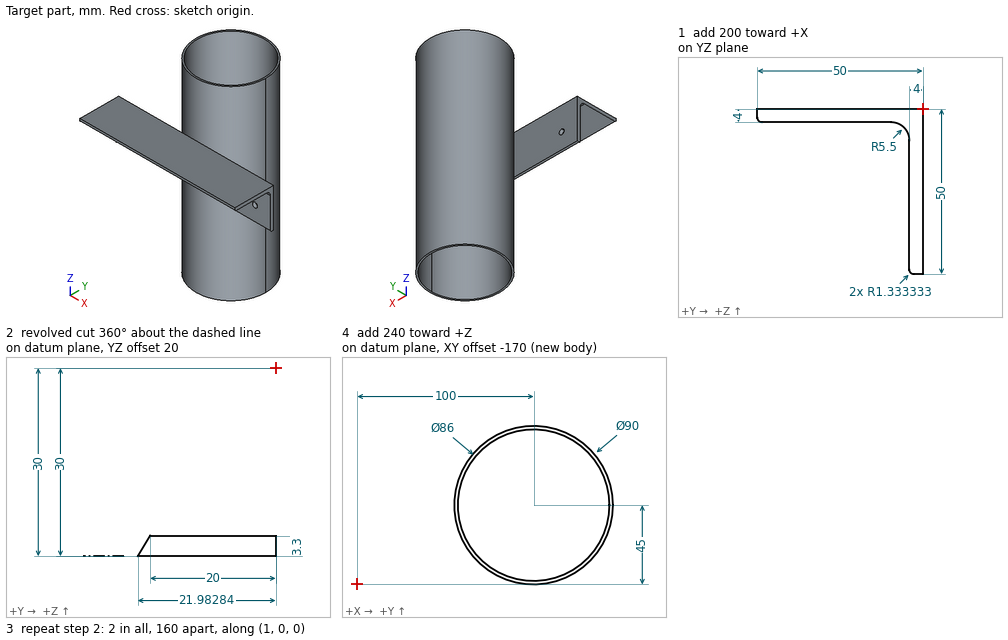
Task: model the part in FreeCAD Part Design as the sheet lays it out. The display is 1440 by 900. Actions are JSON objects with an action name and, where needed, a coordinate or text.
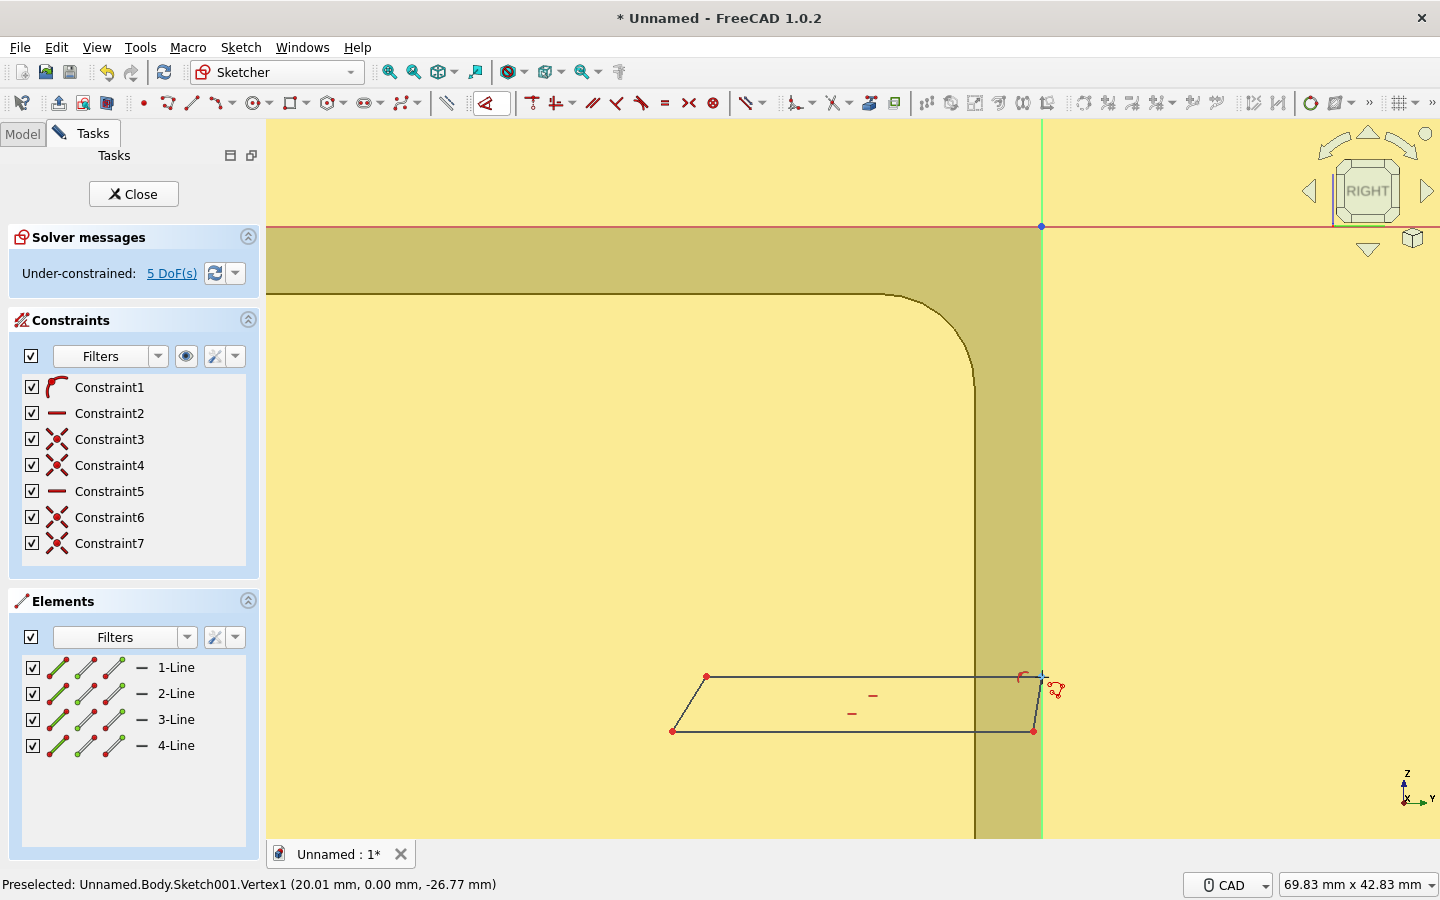
{"action": "left_click", "coordinate": [192, 104]}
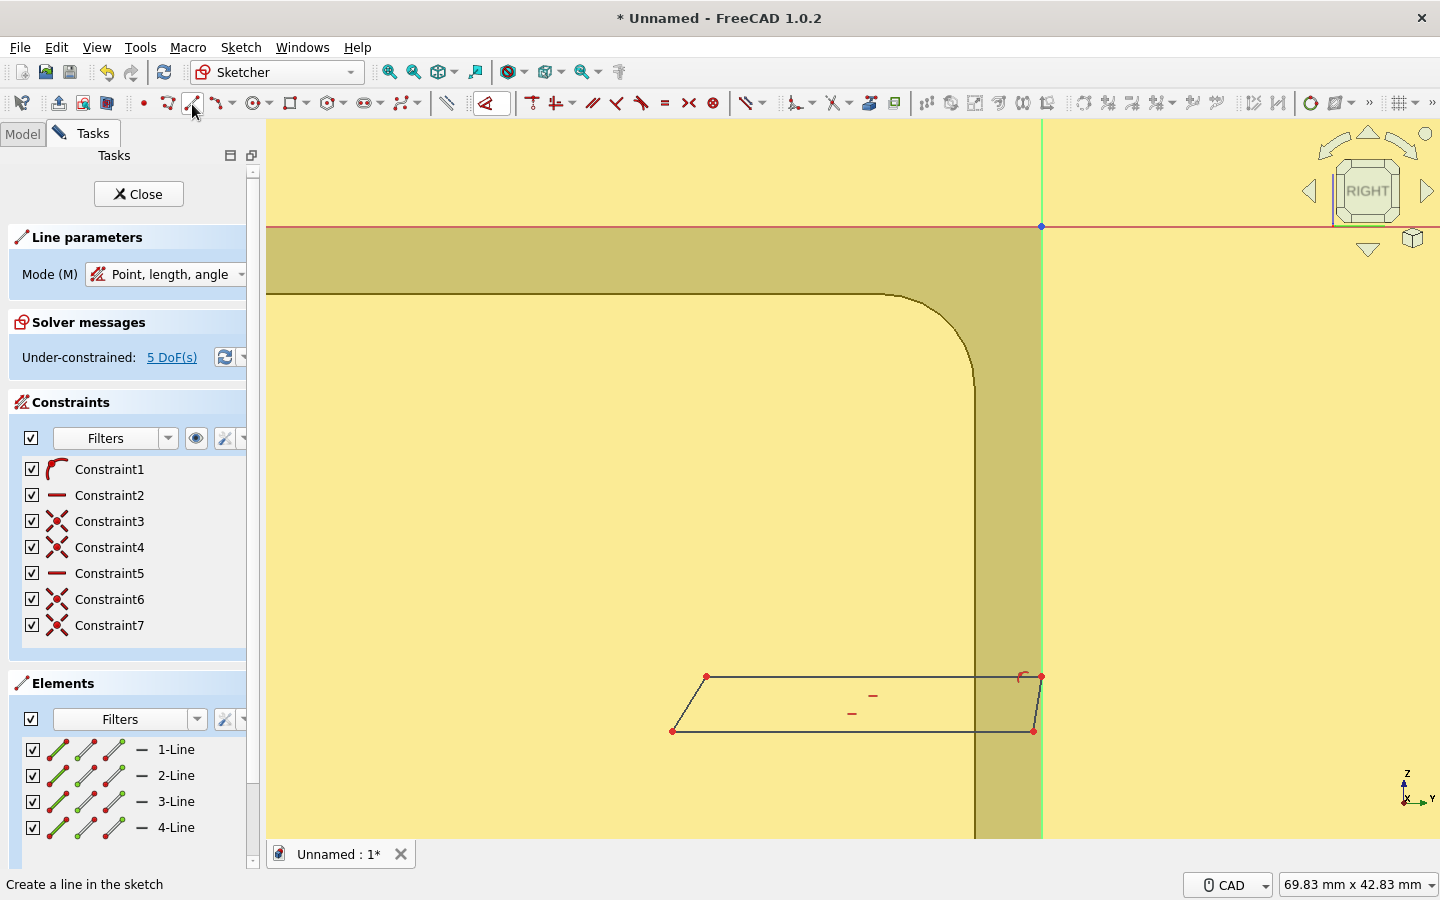
{"action": "left_click", "coordinate": [635, 731]}
{"action": "left_click", "coordinate": [524, 731]}
{"action": "key", "text": "Escape"}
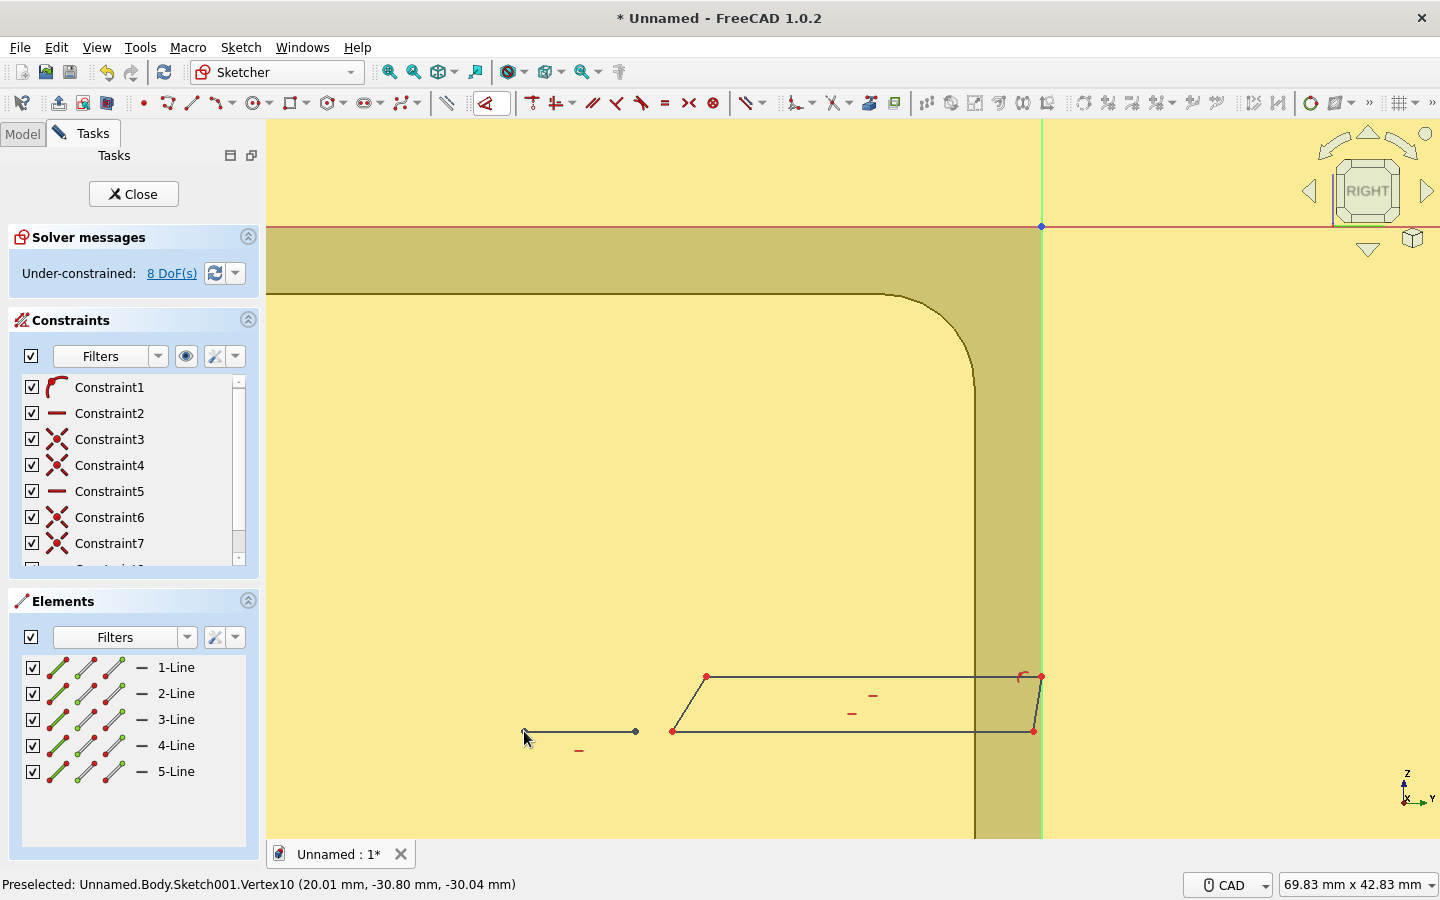
{"action": "left_click", "coordinate": [602, 732]}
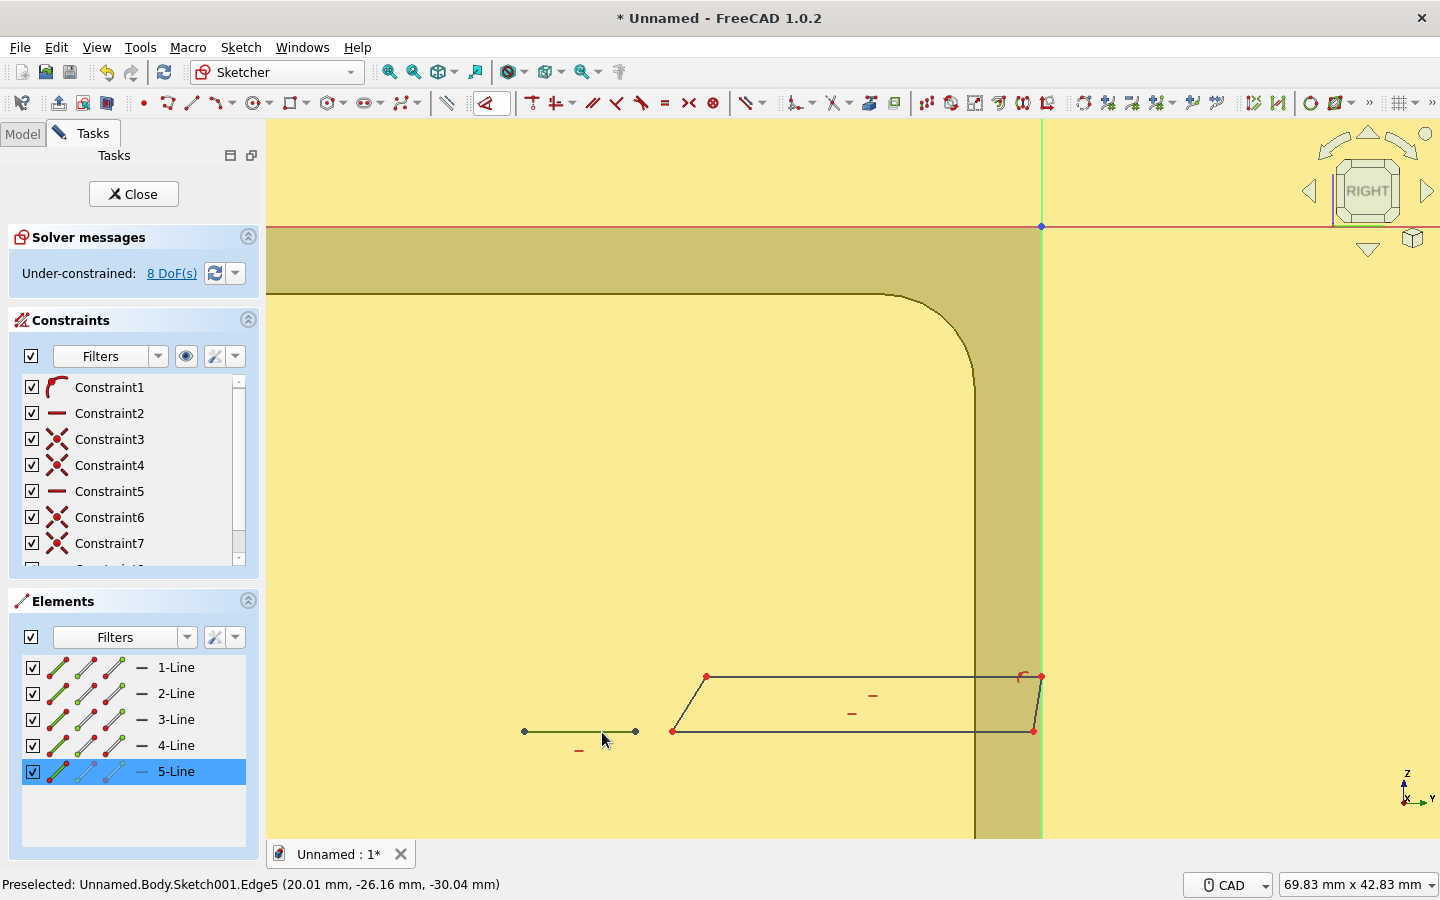
{"action": "left_click", "coordinate": [448, 104]}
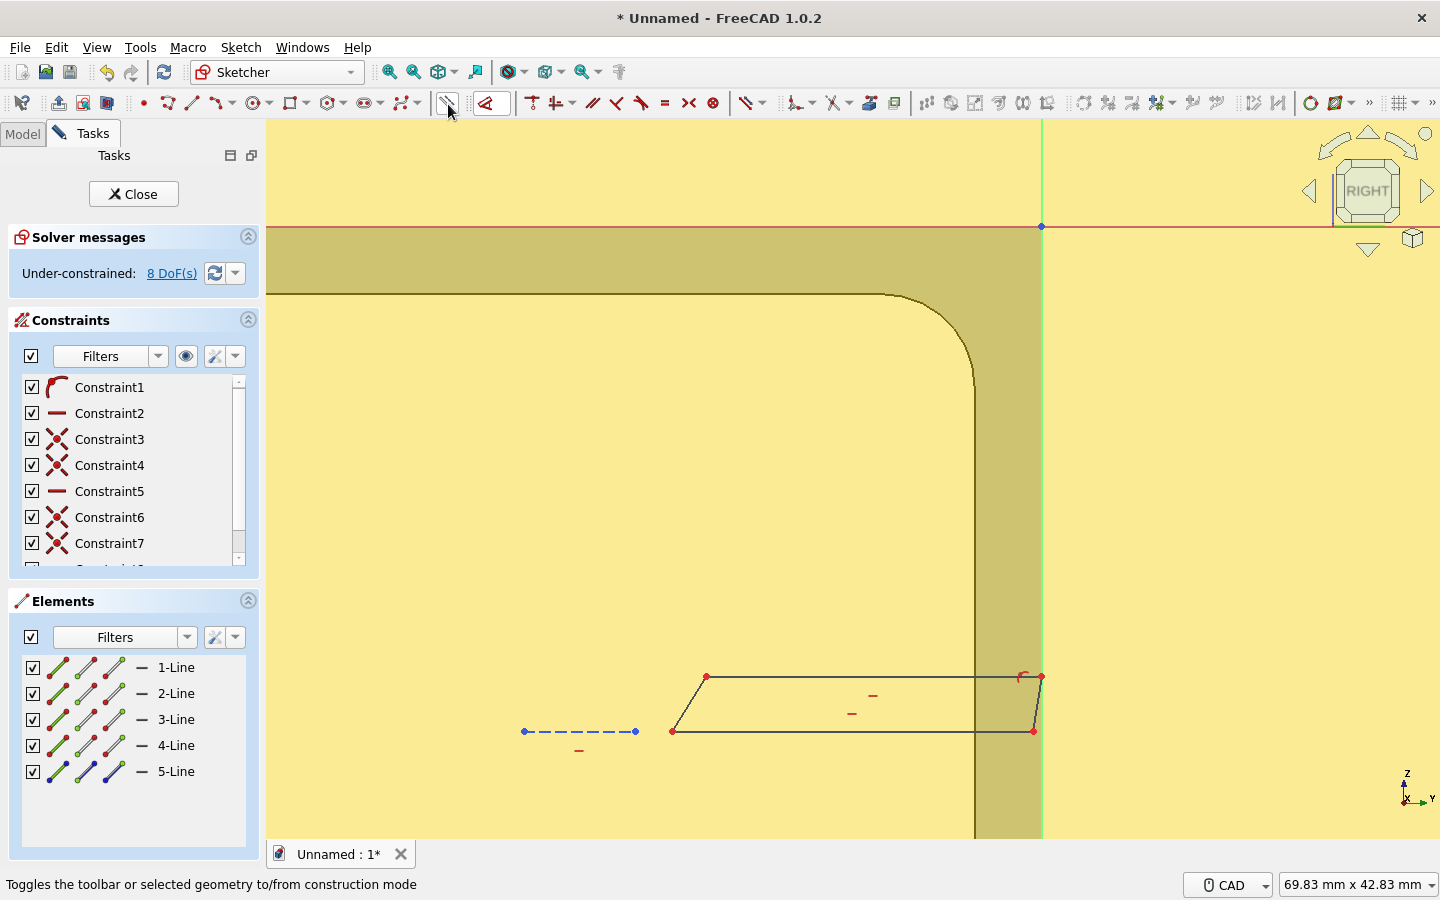
{"action": "left_click", "coordinate": [1039, 694]}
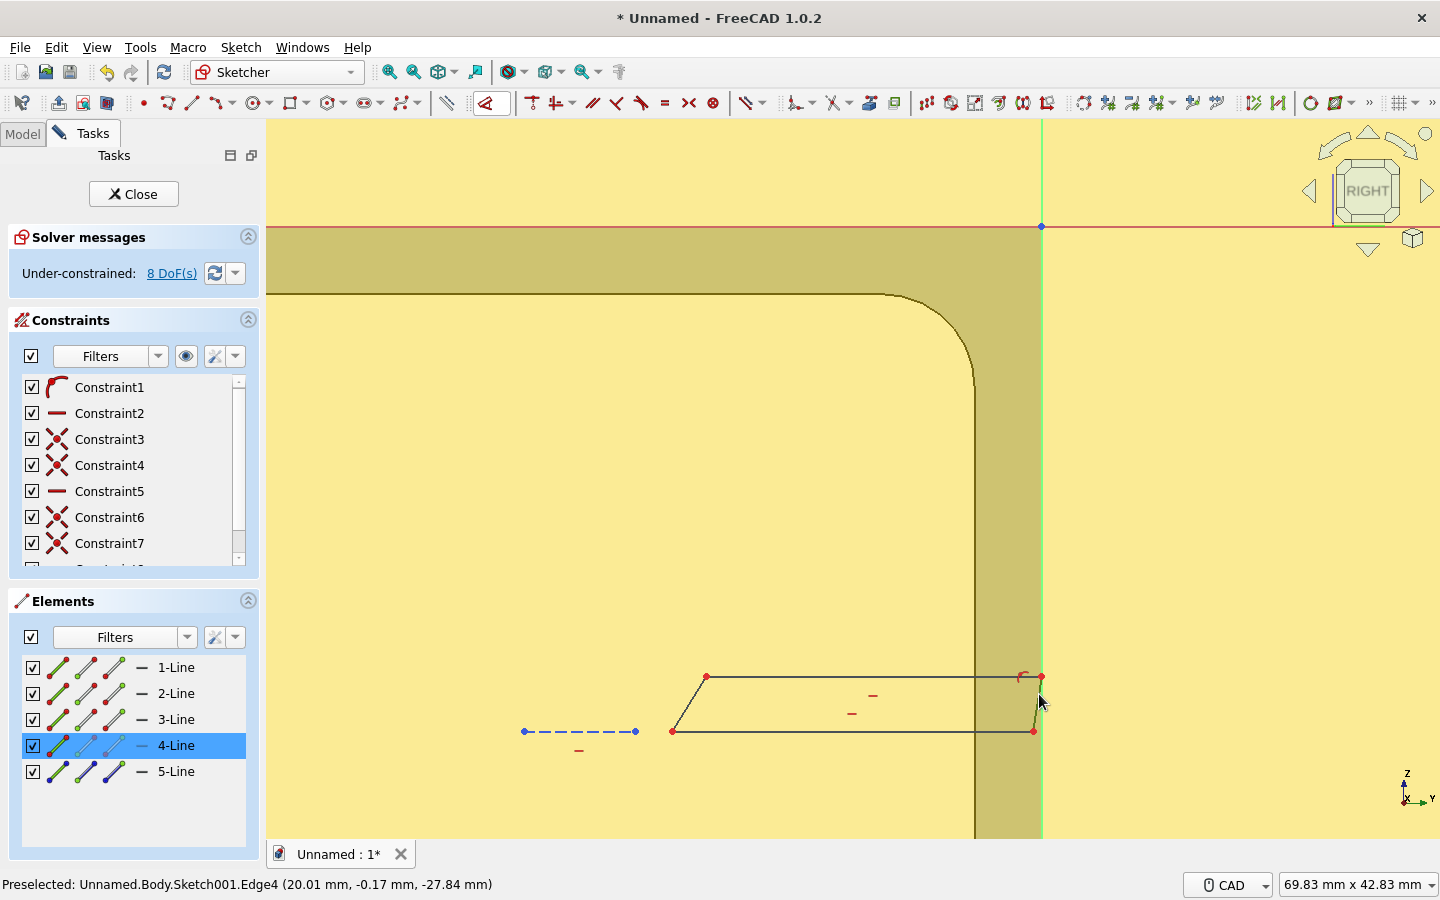
{"action": "left_click", "coordinate": [574, 104]}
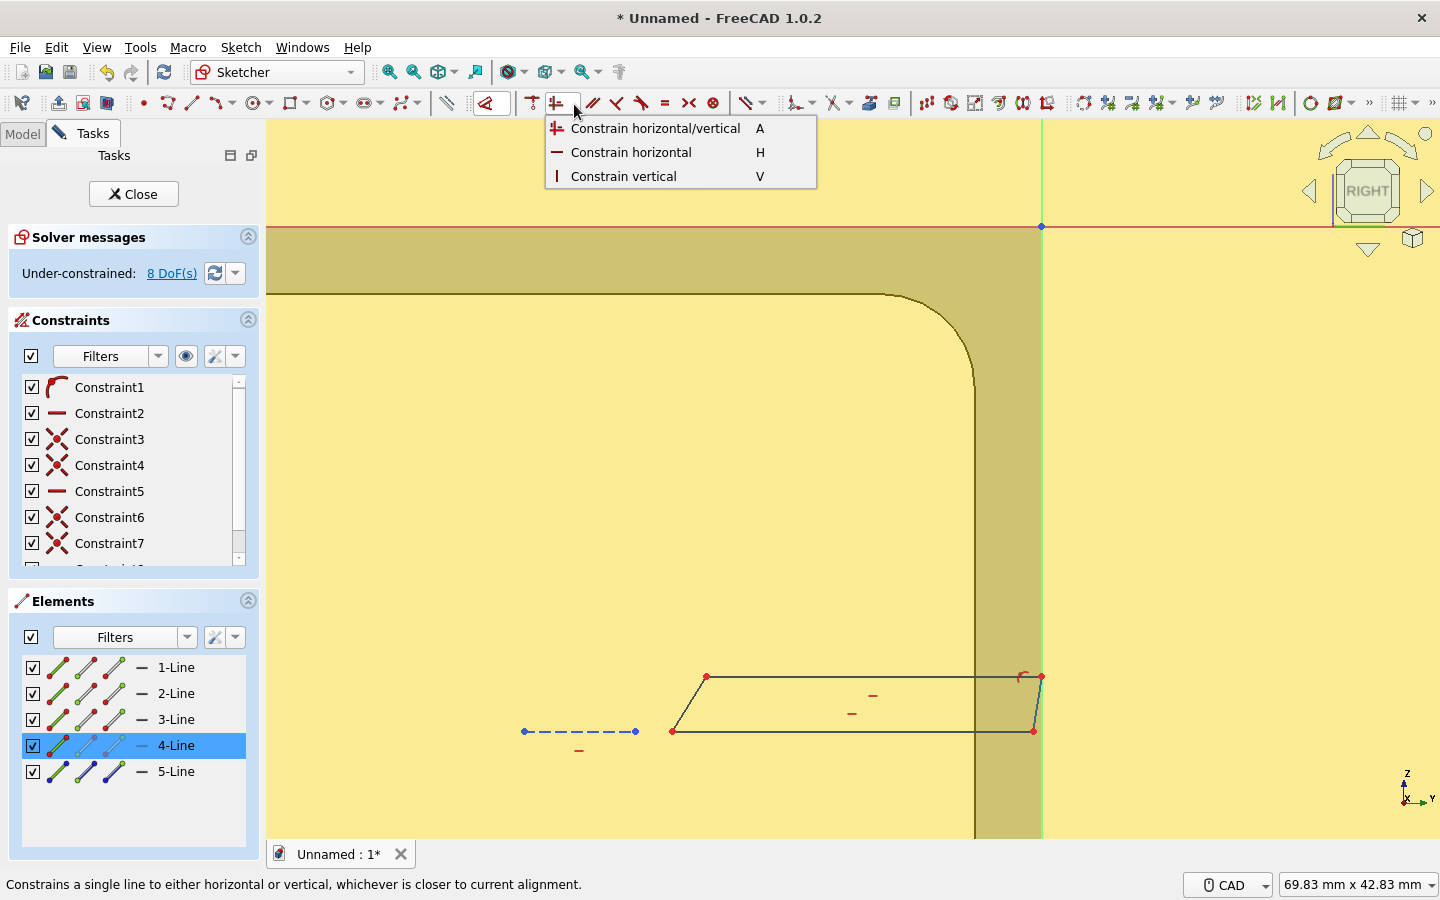
{"action": "left_click", "coordinate": [681, 176]}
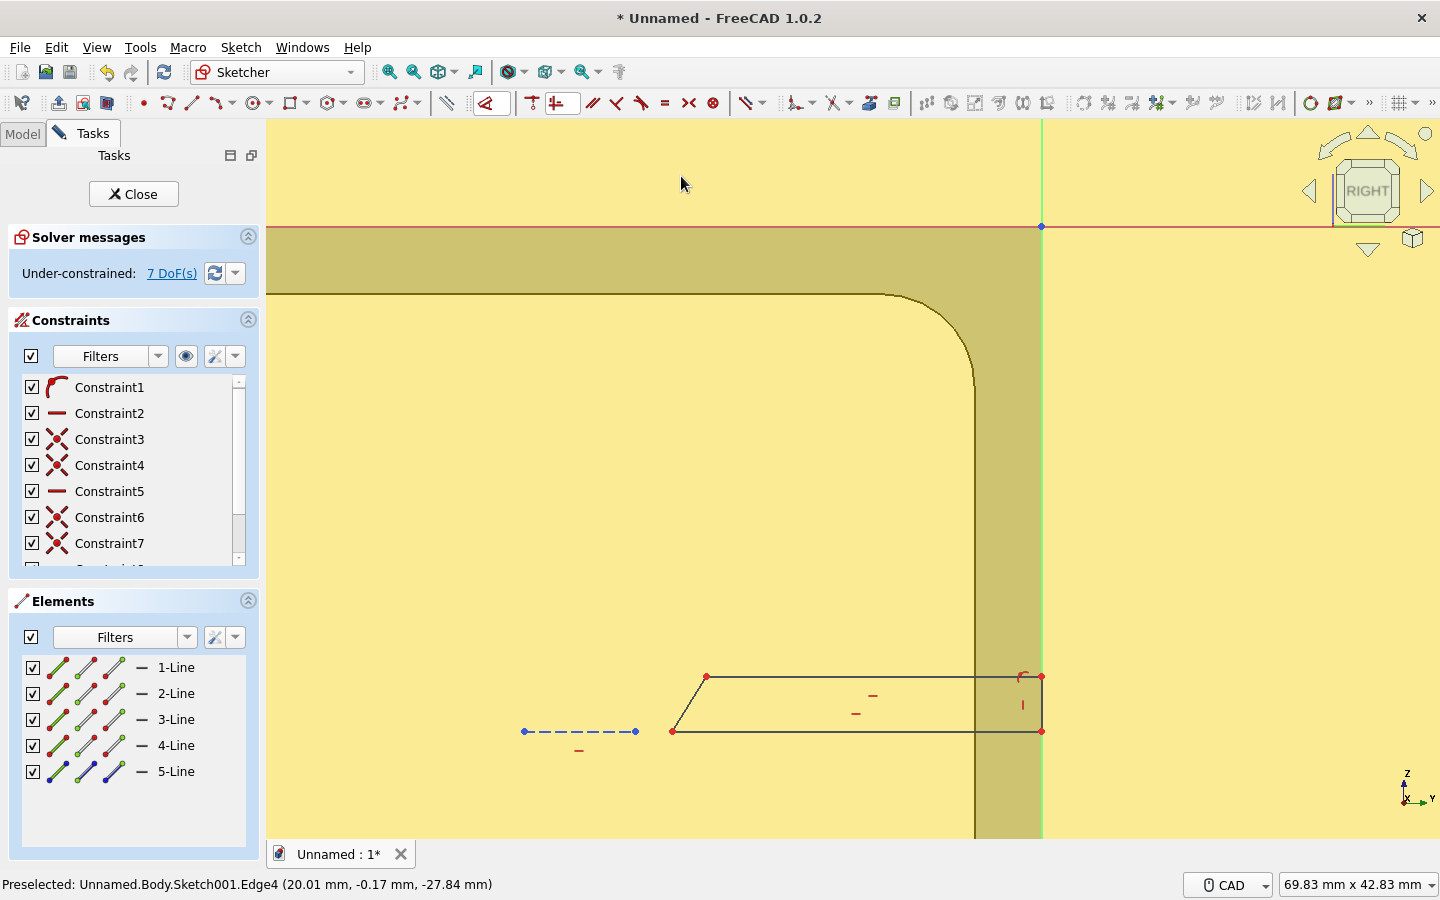
{"action": "left_click", "coordinate": [941, 677]}